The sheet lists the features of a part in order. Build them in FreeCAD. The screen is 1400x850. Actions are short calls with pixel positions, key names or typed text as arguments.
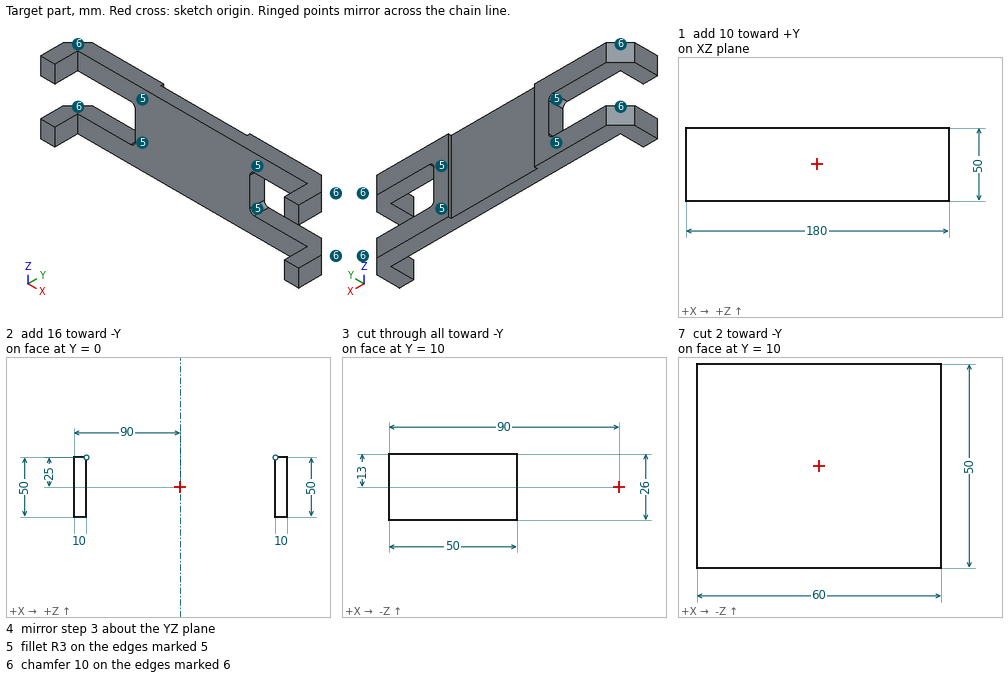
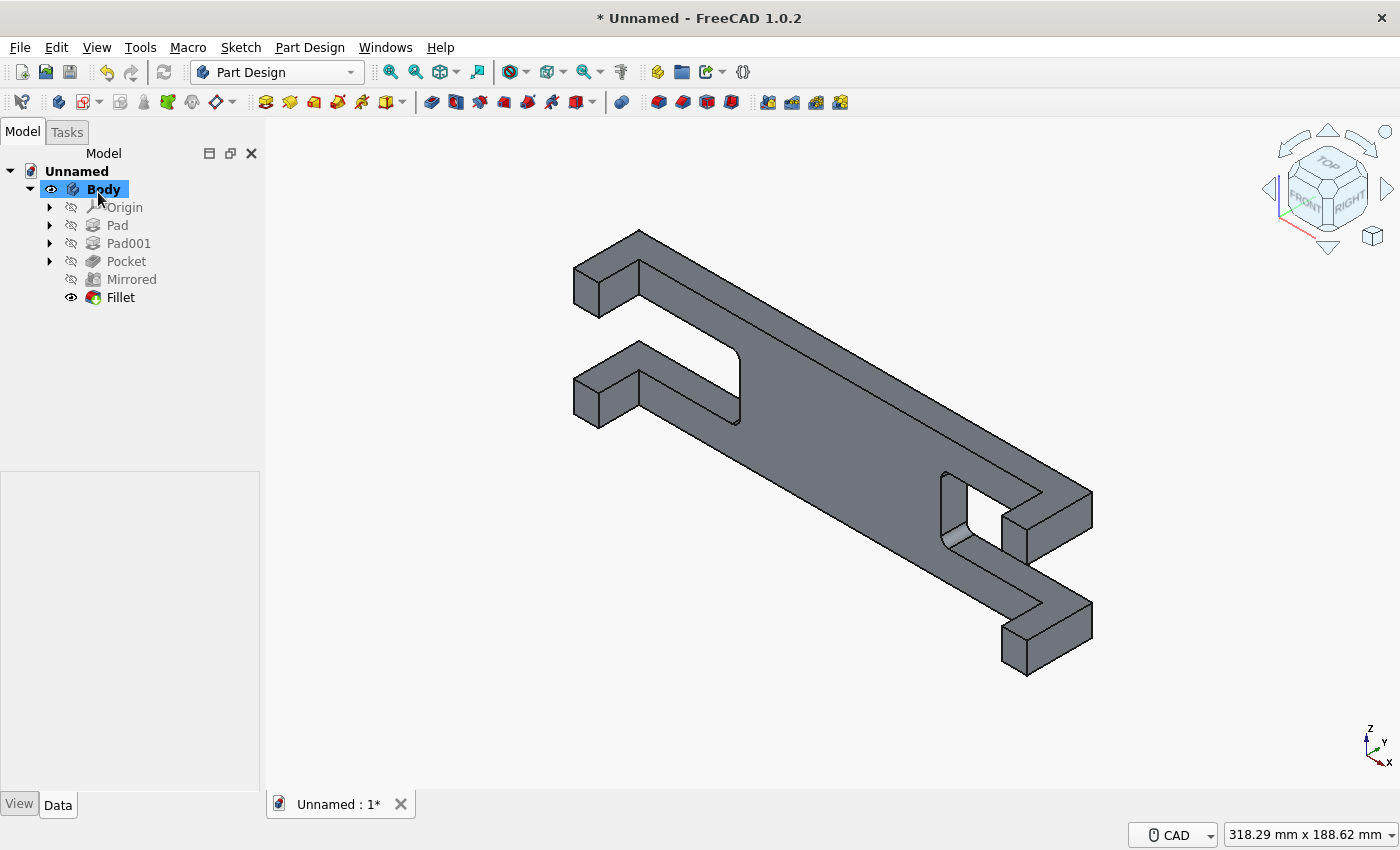
key(1)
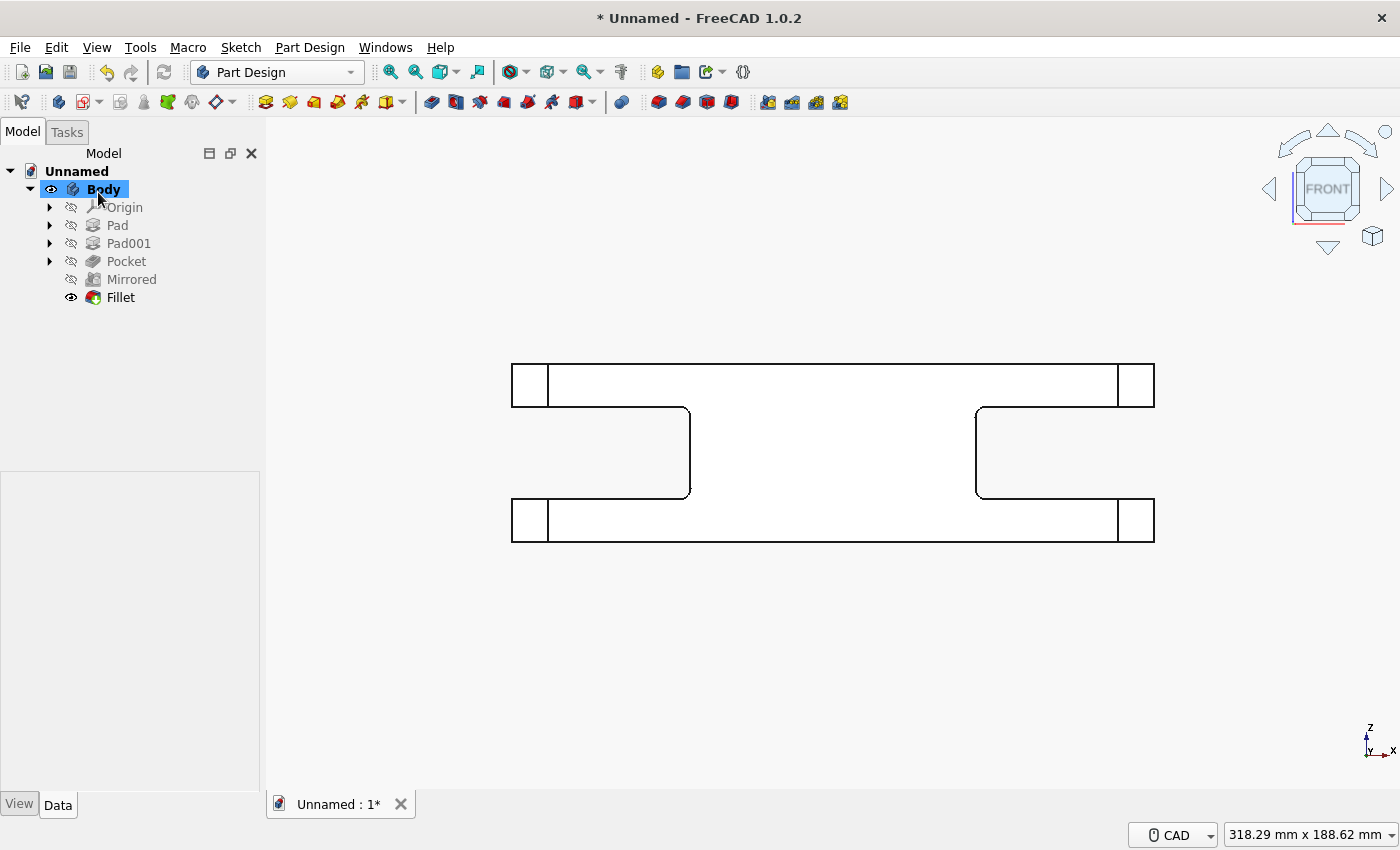
key(3)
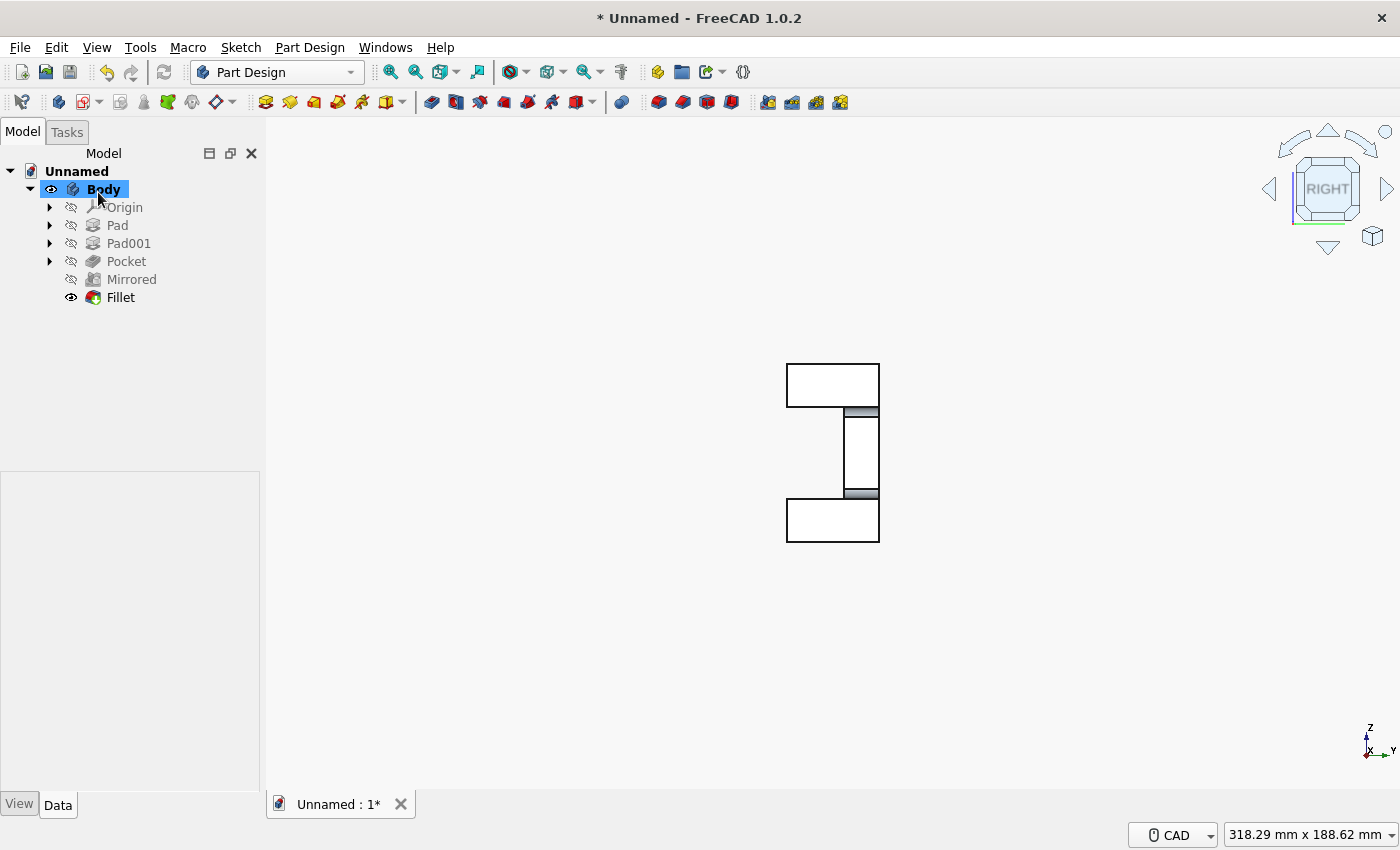
key(v)
key(f)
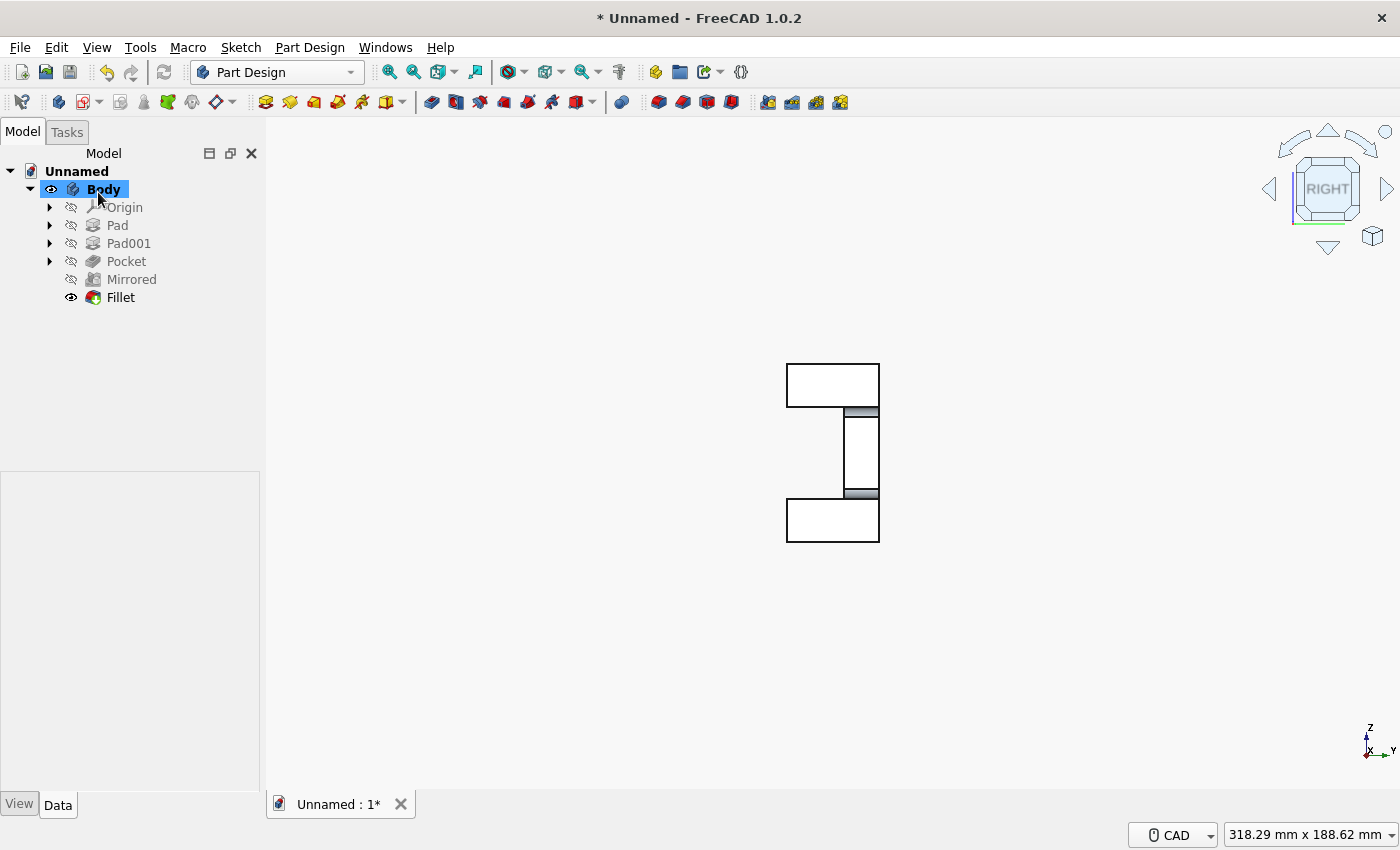
click(879, 384)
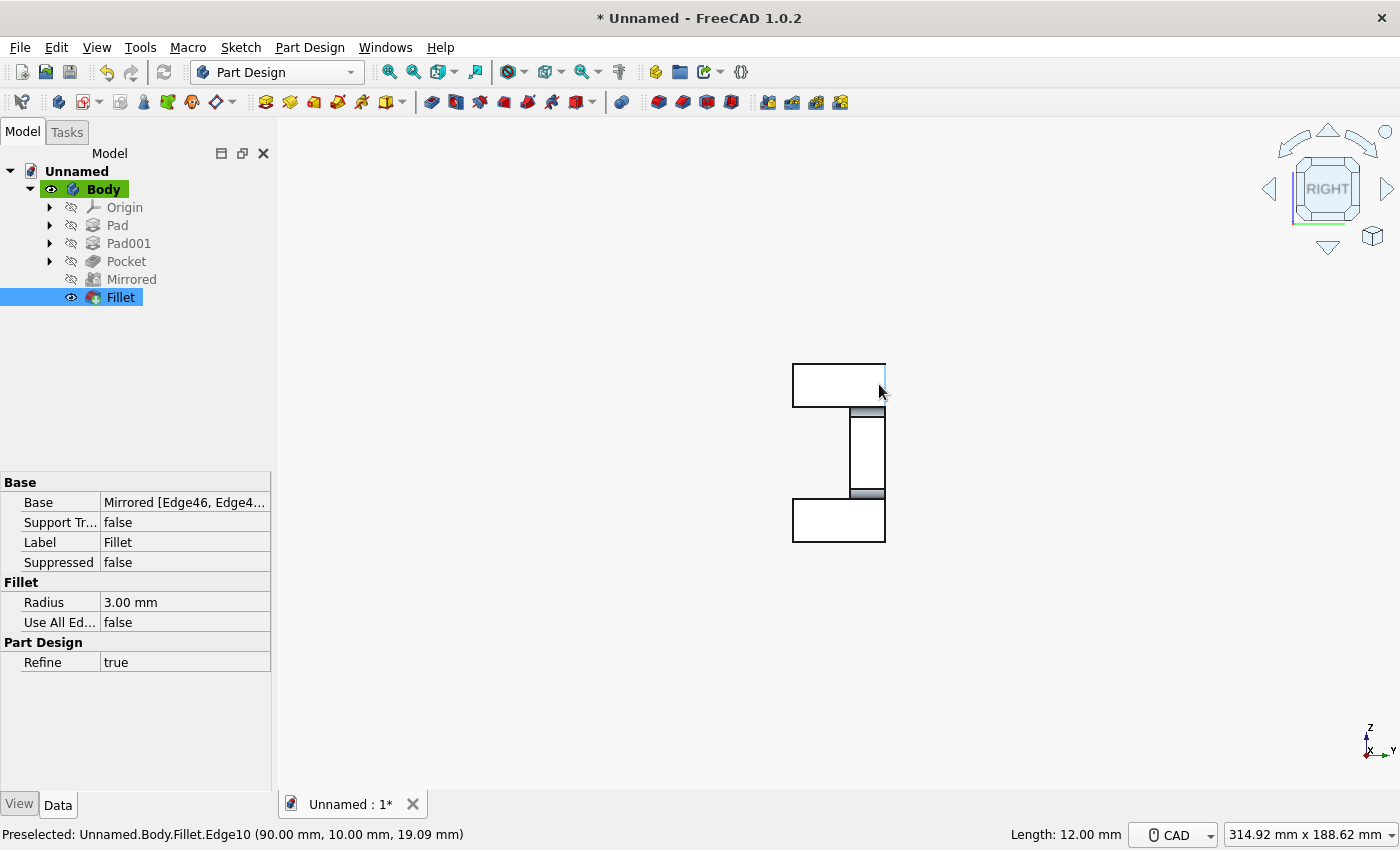
click(885, 520, ctrl)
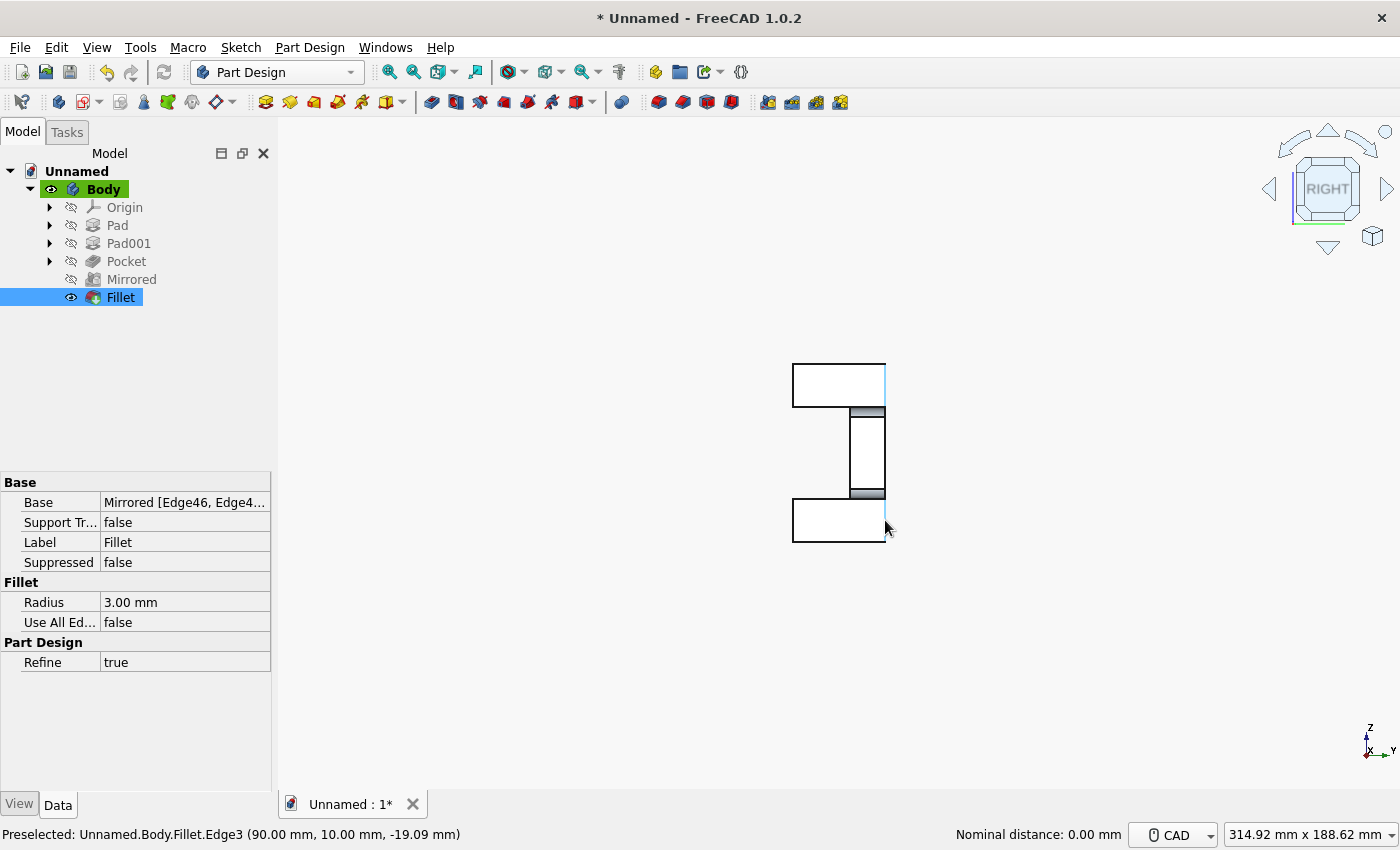
key(5)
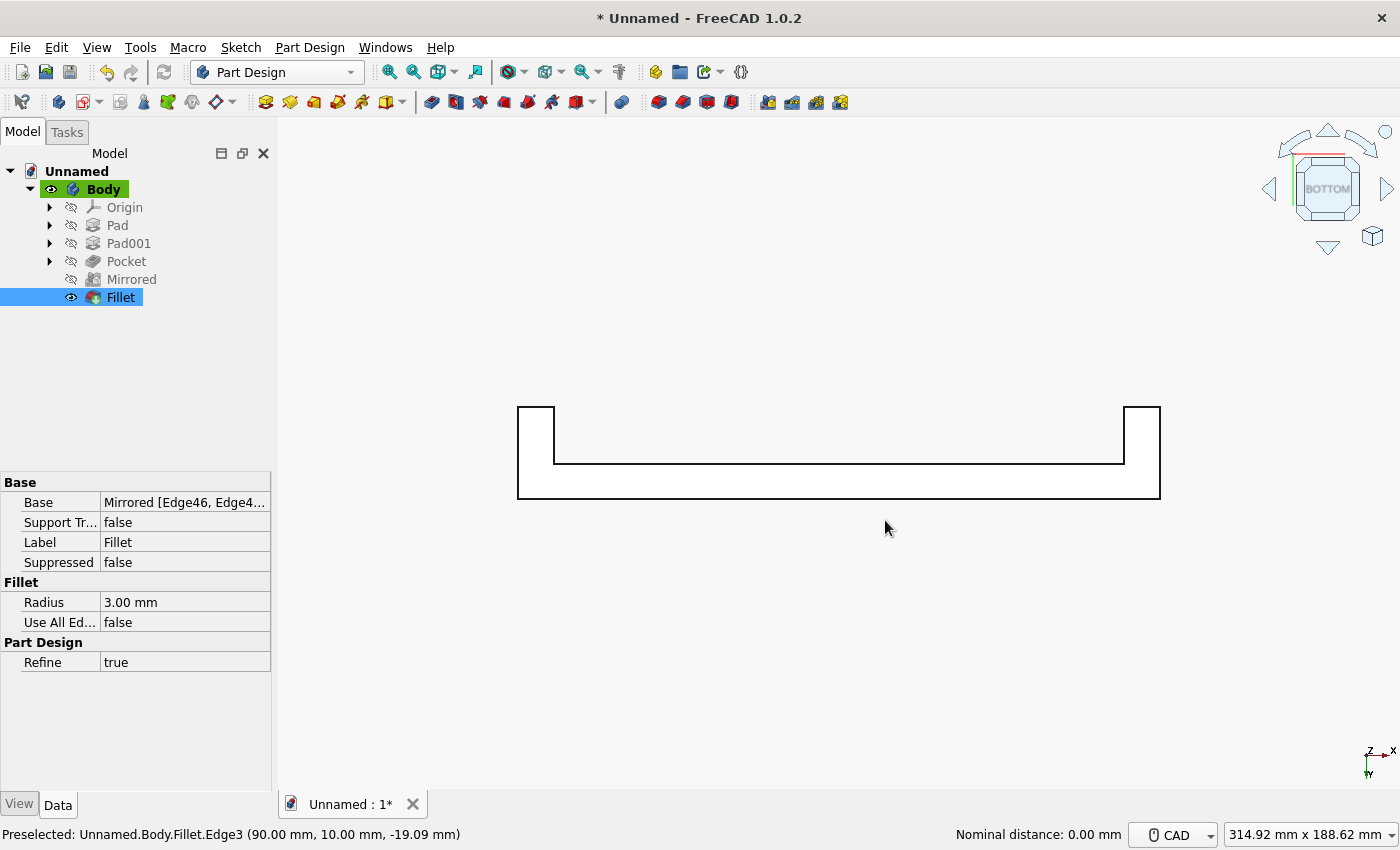
key(4)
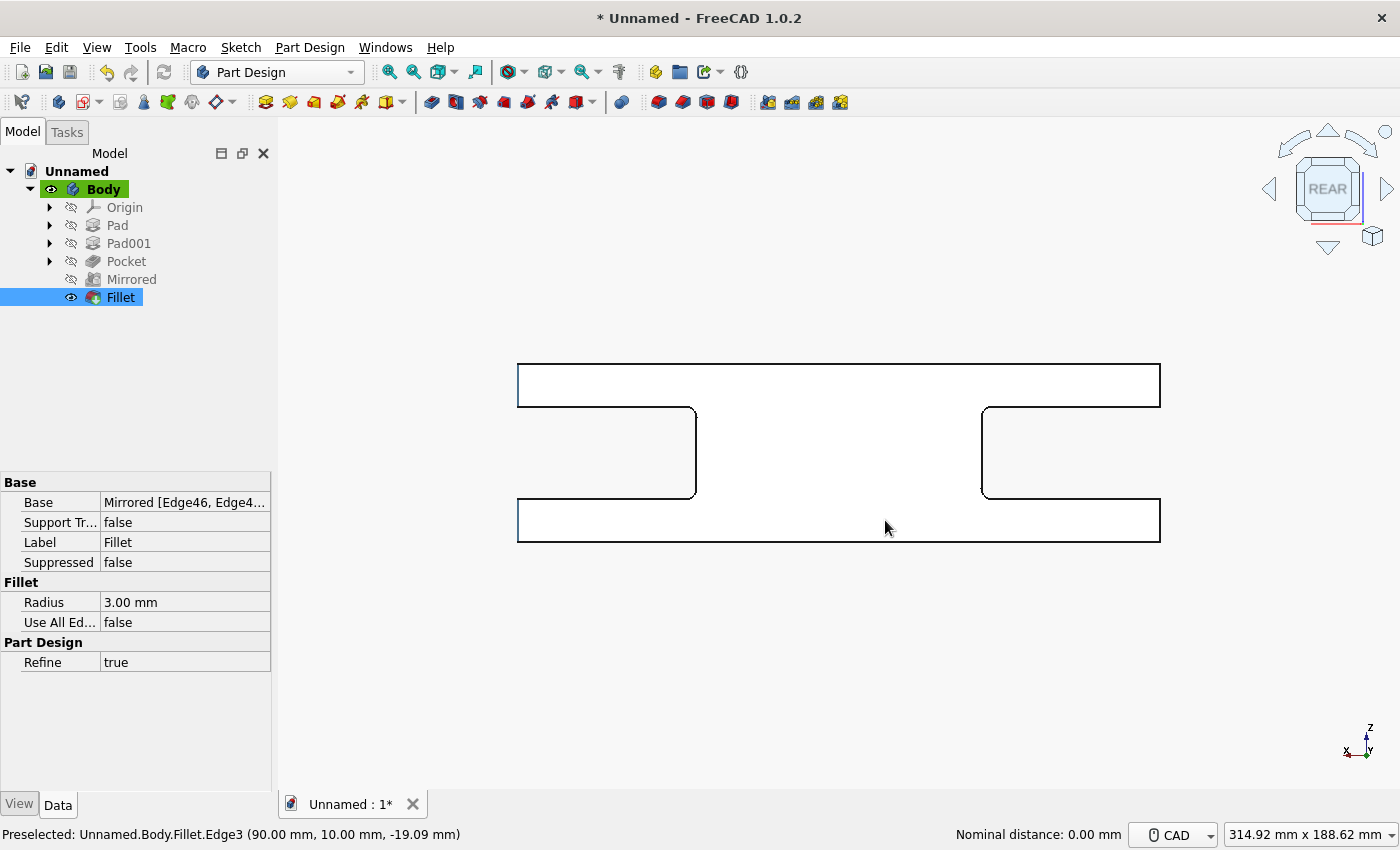
click(1160, 520, ctrl)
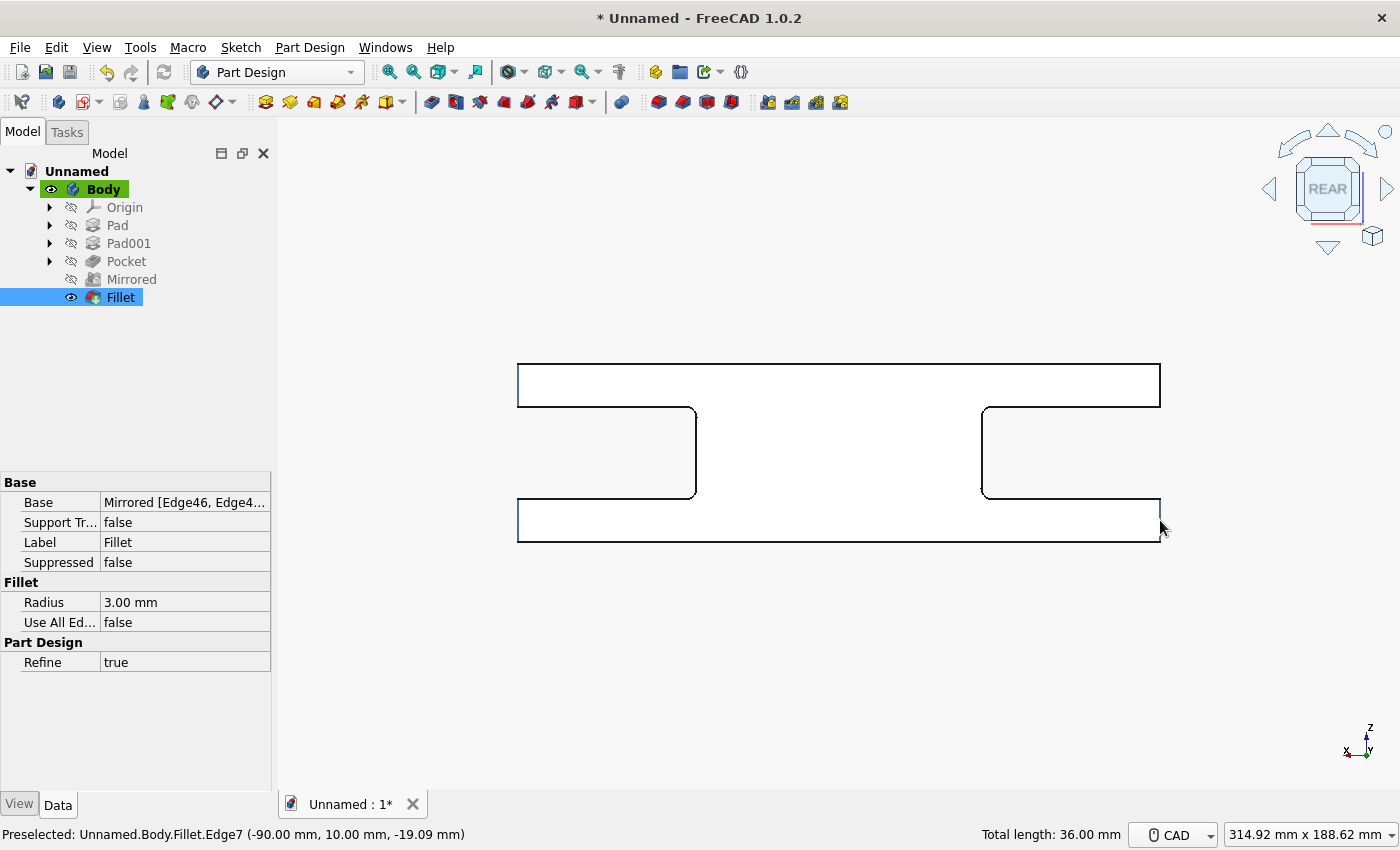
click(1160, 384, ctrl)